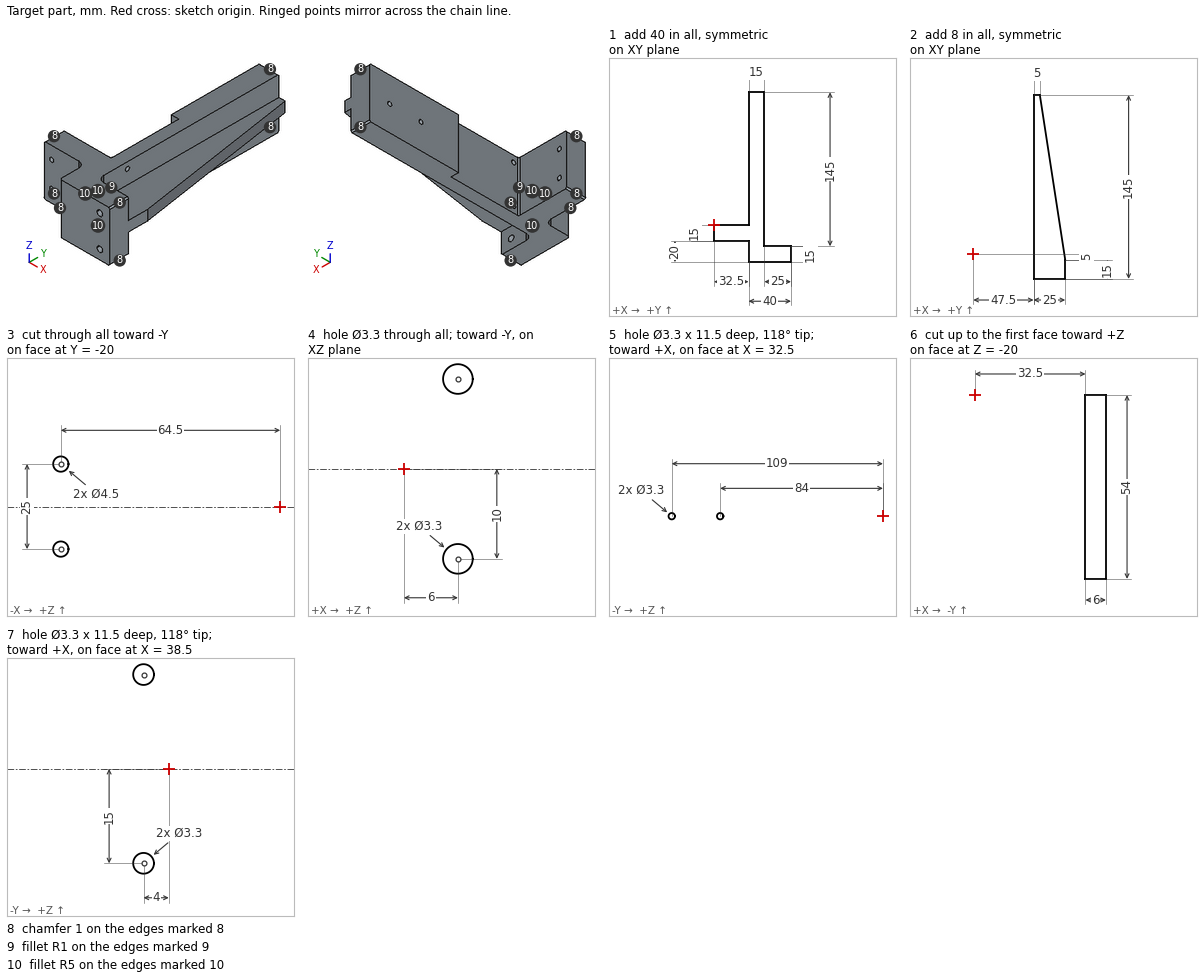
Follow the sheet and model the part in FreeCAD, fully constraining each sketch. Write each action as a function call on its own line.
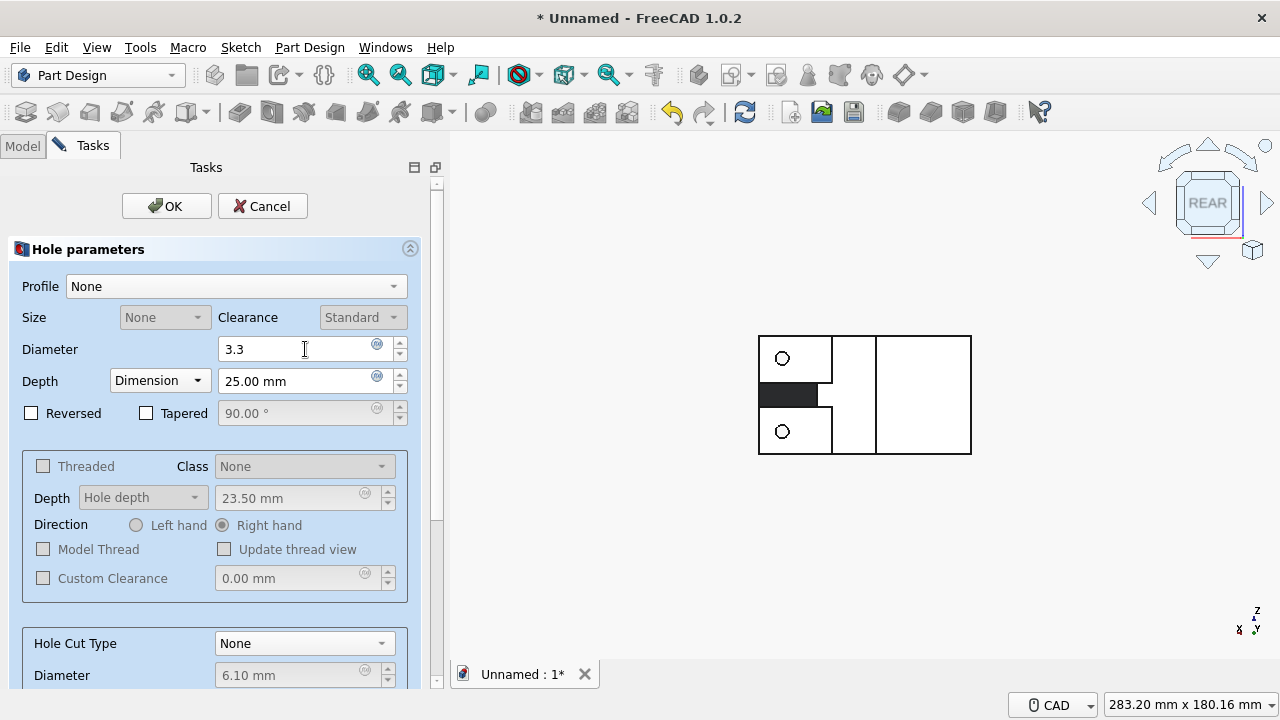
click(161, 380)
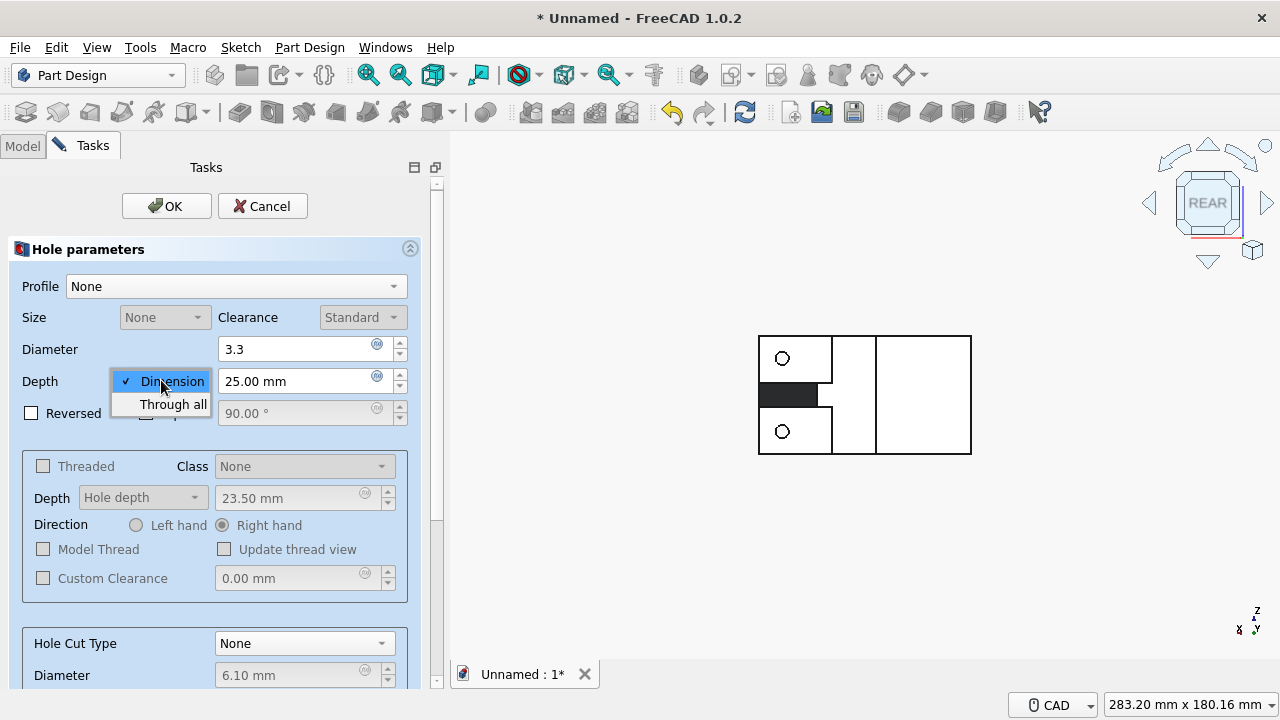
click(160, 404)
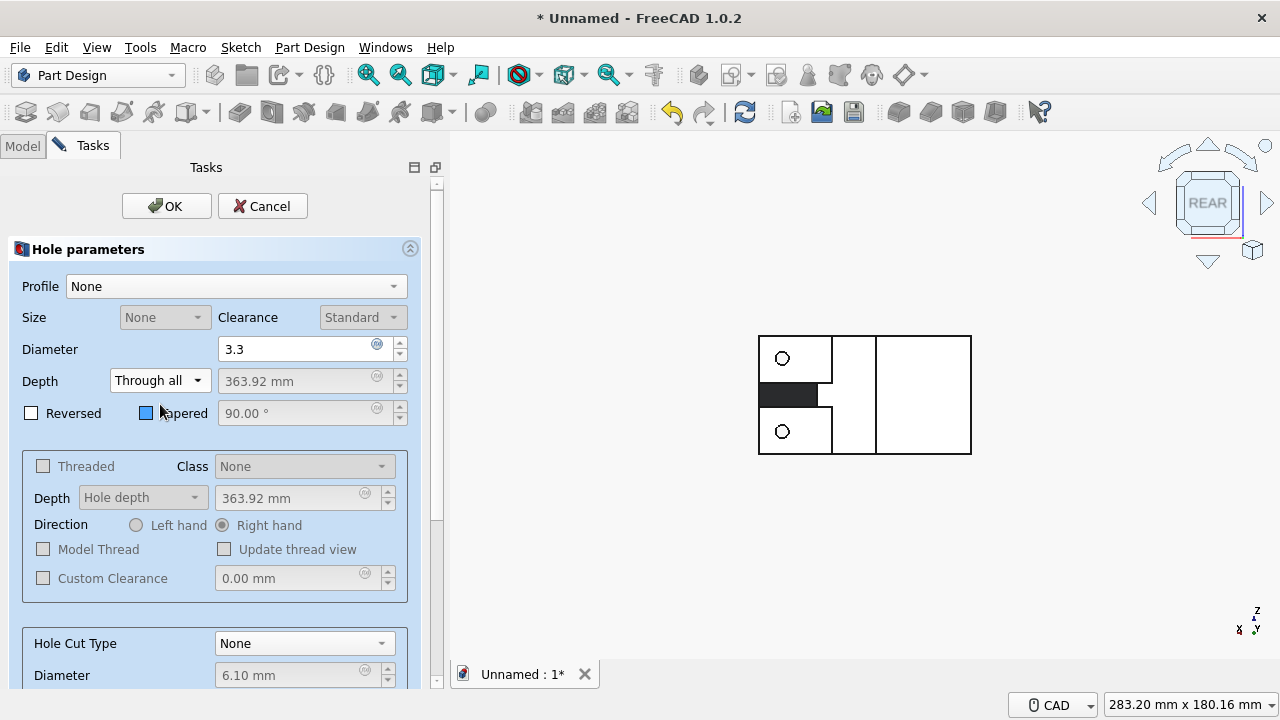
click(30, 413)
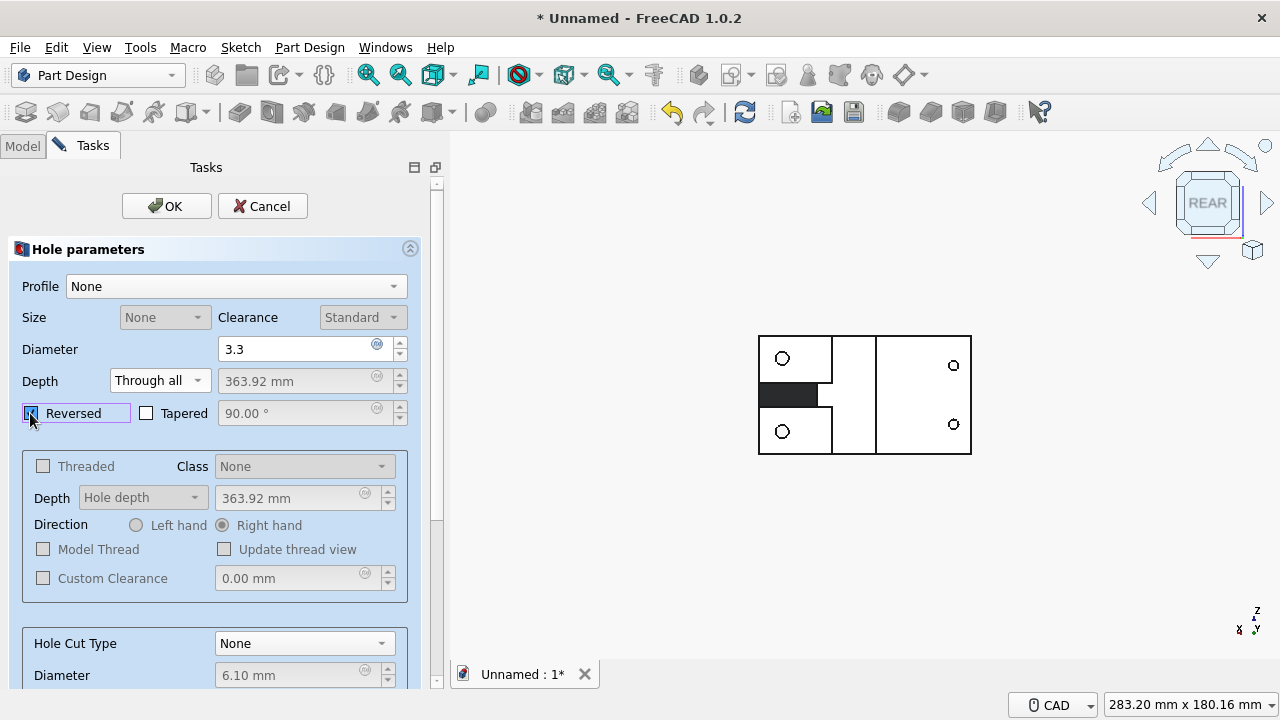
click(167, 206)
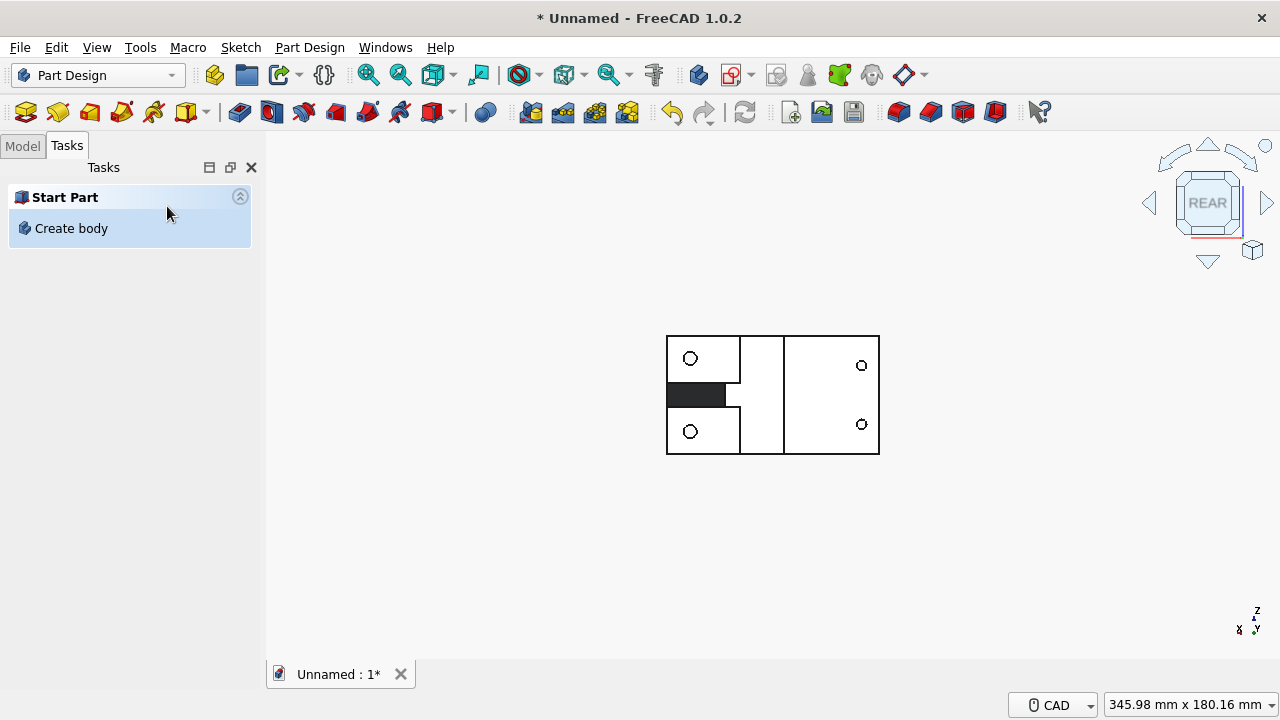
click(370, 76)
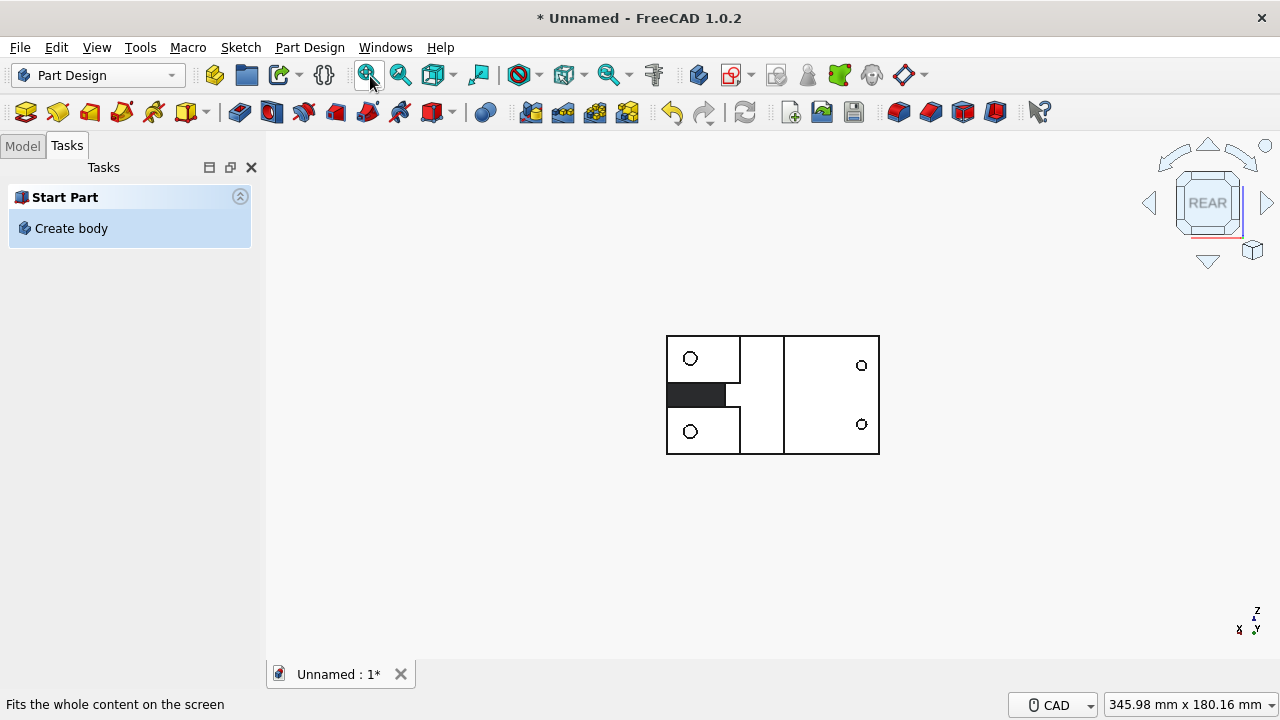
key(6)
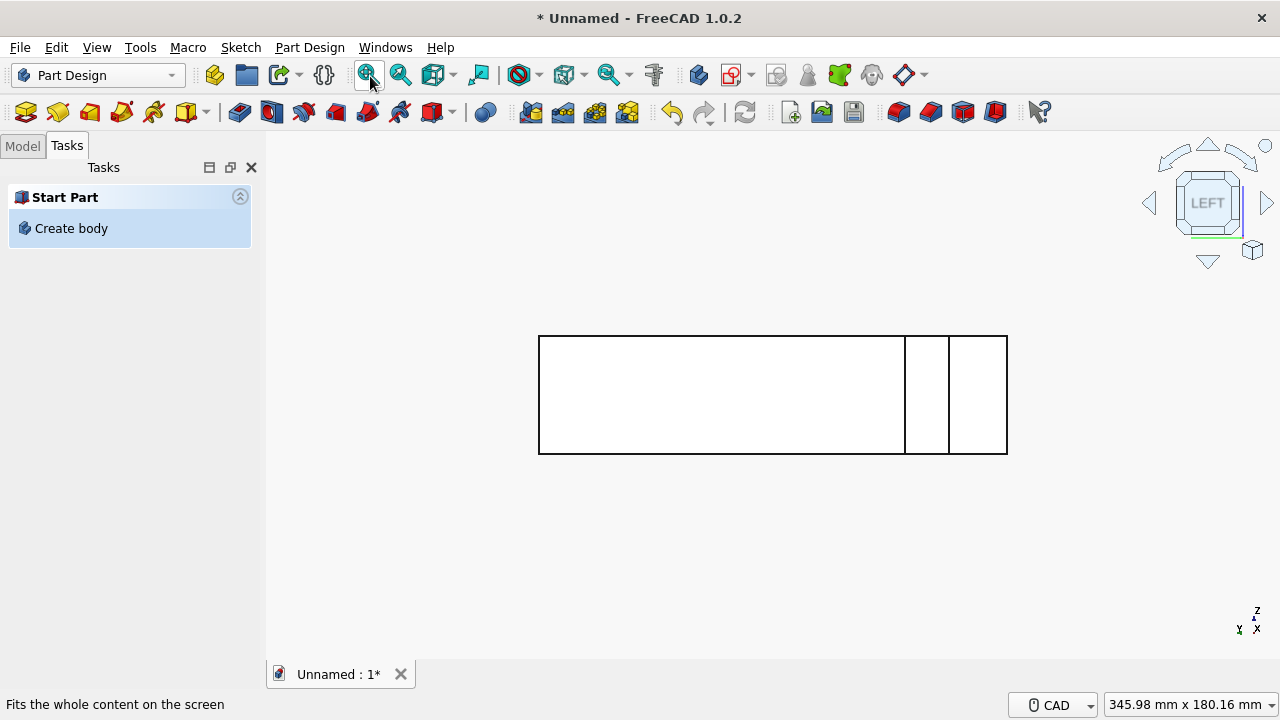
click(617, 394)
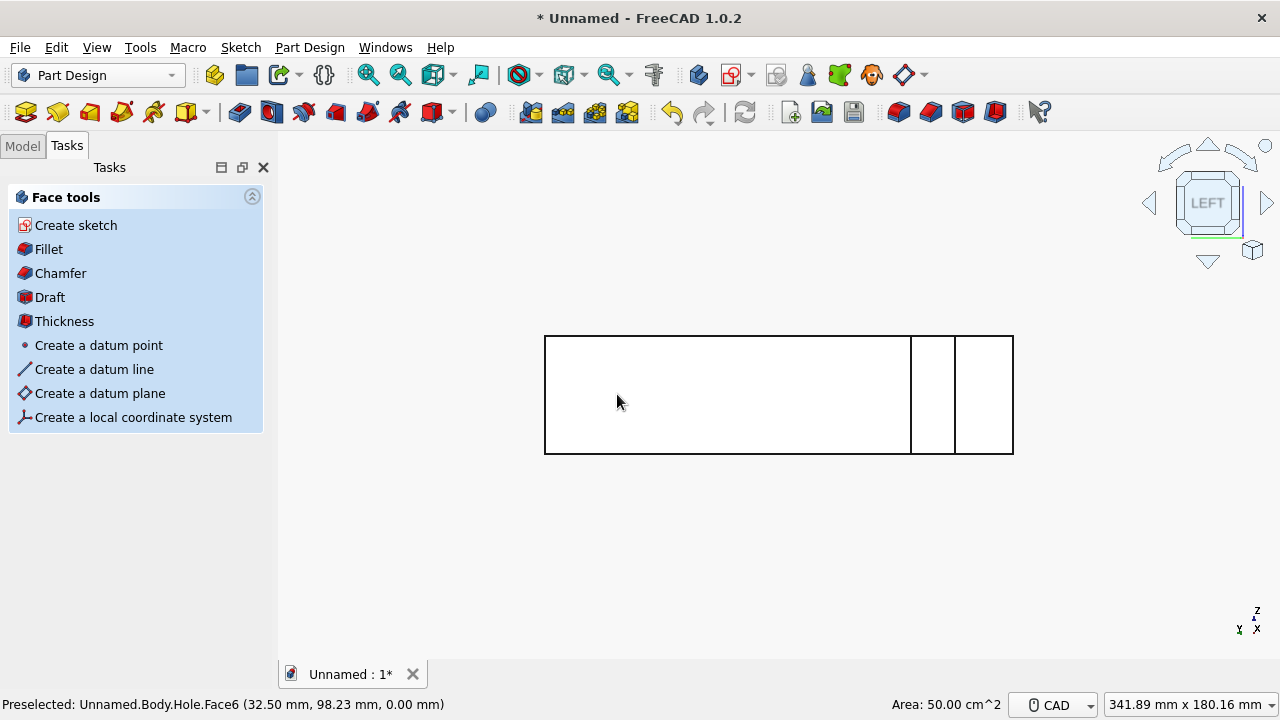
click(732, 76)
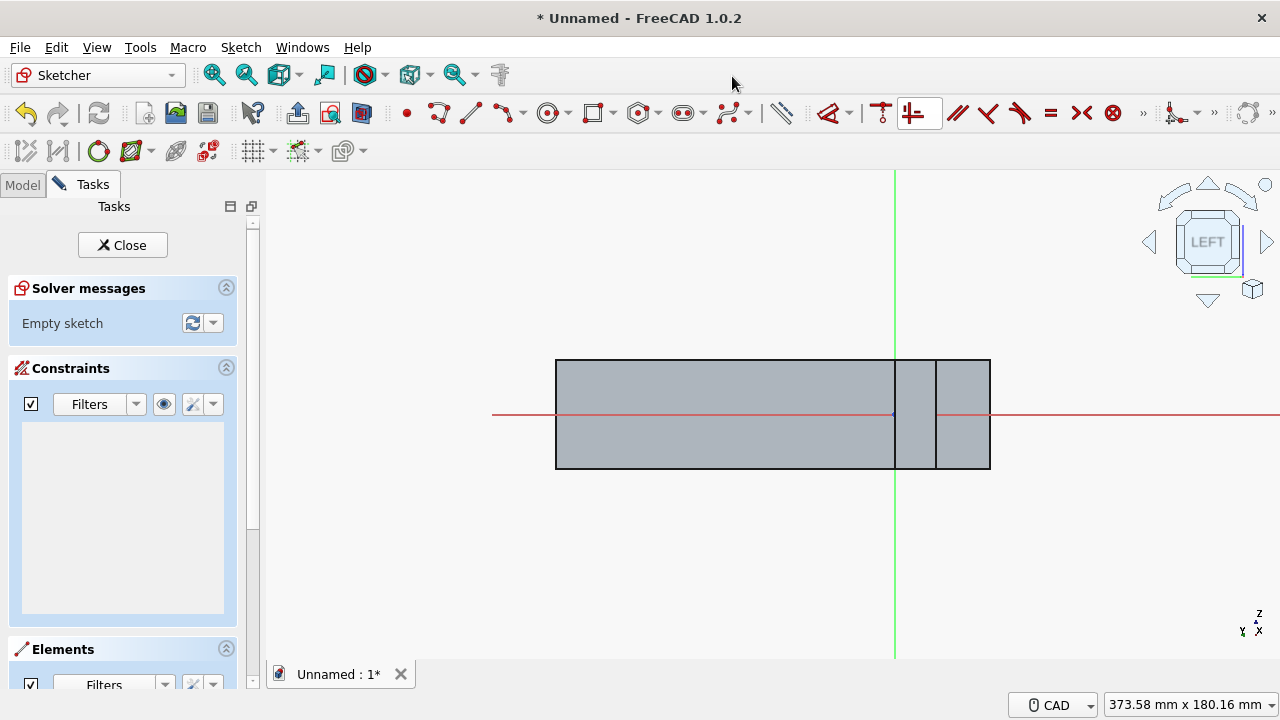
scroll(622, 414, up, 10)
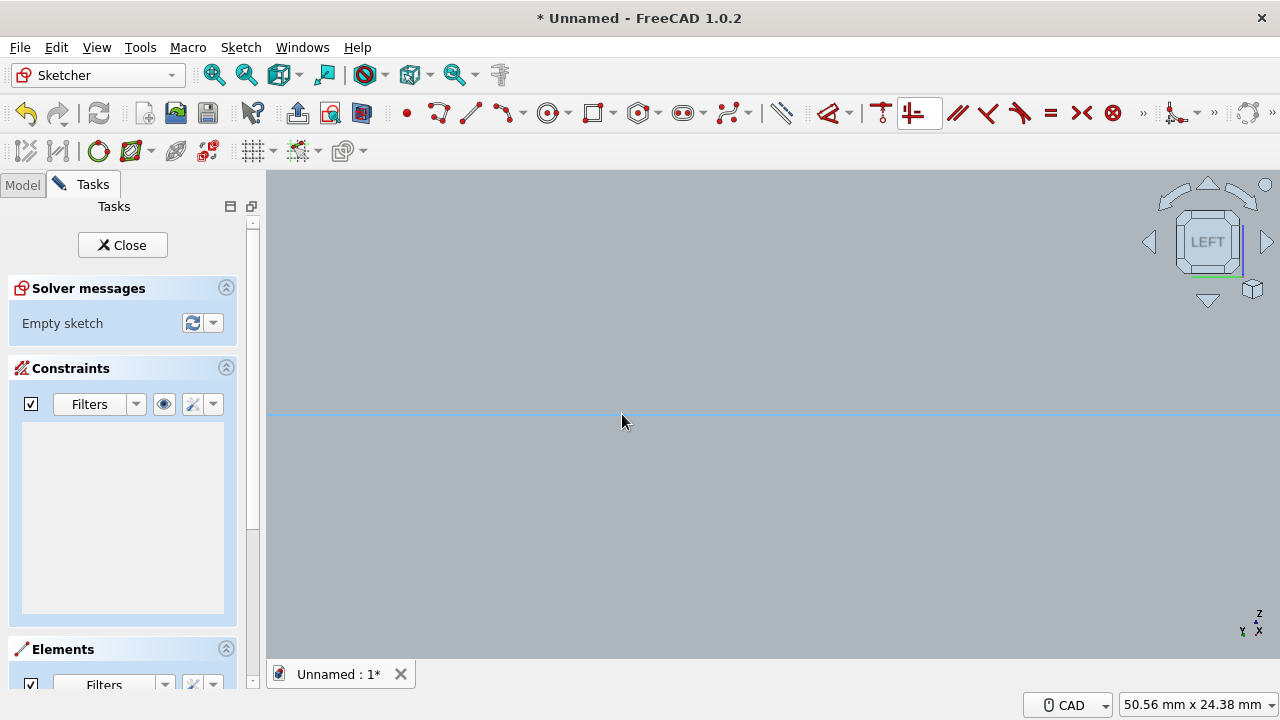
click(548, 114)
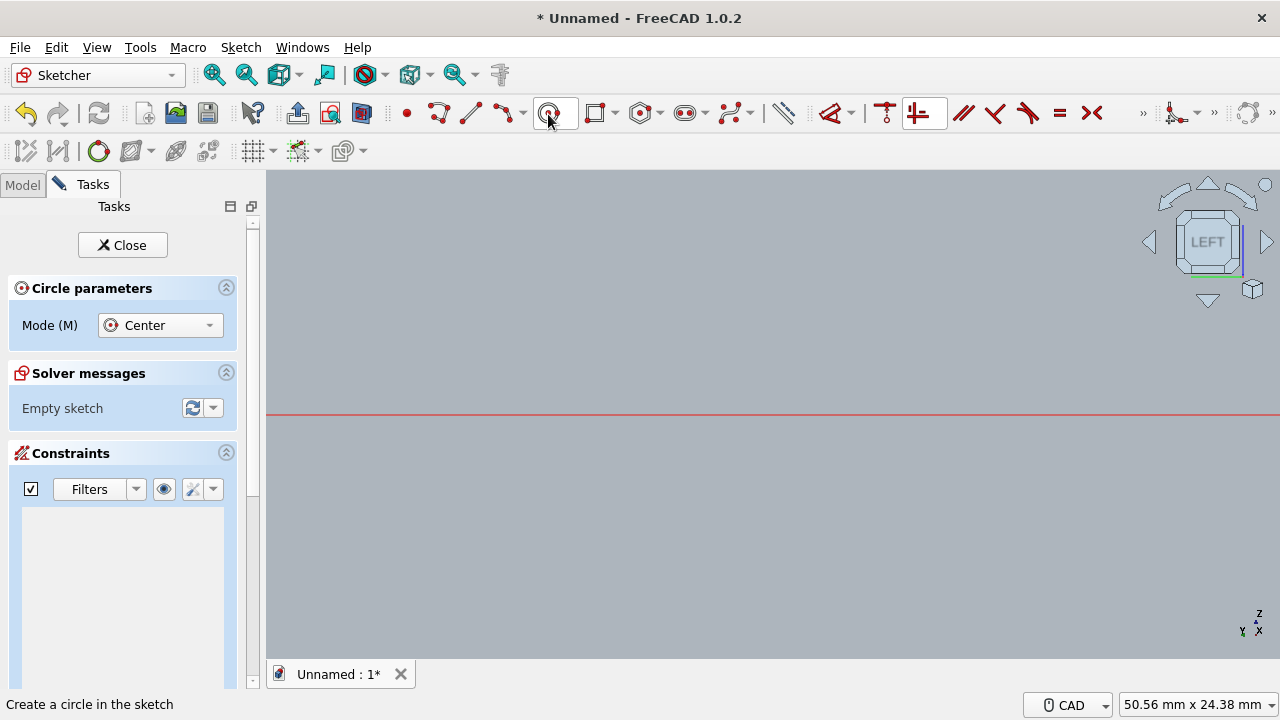
click(452, 414)
click(475, 391)